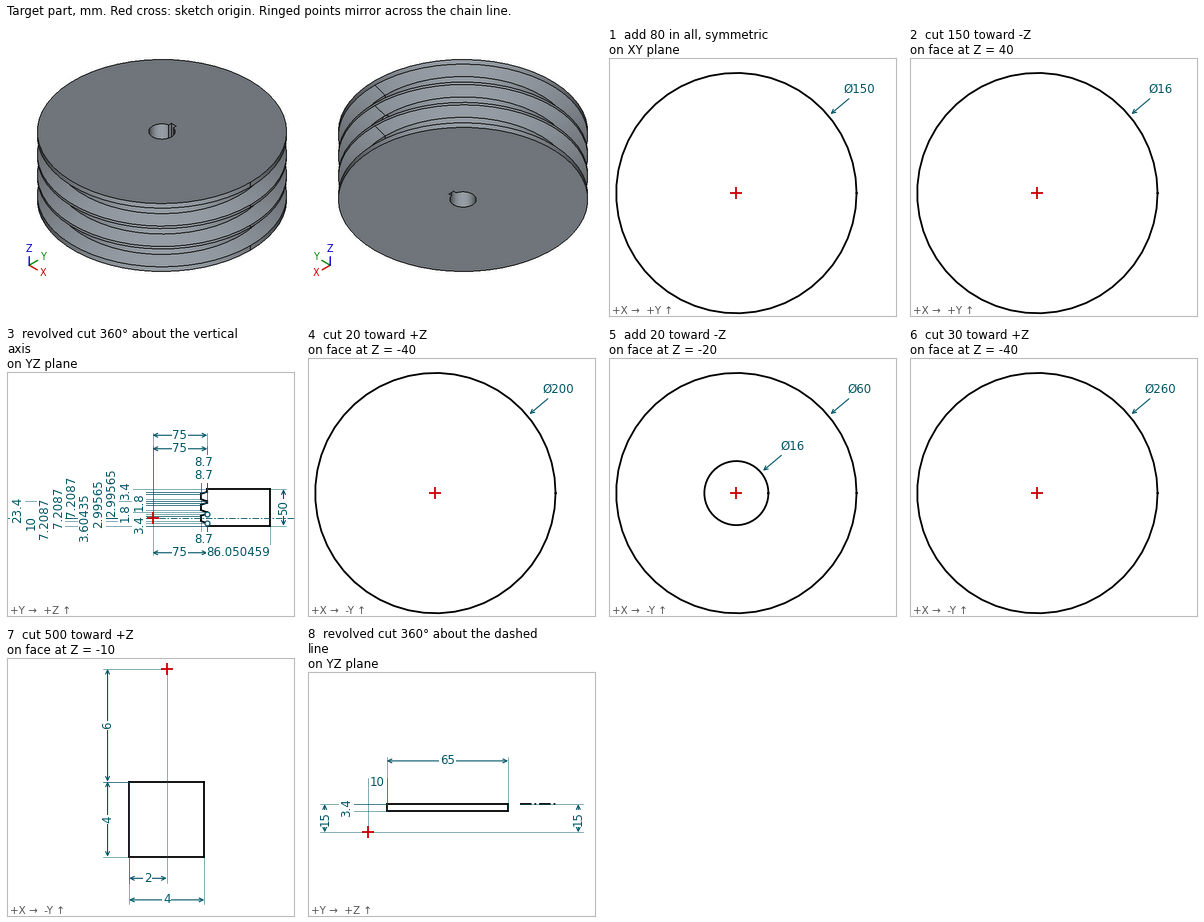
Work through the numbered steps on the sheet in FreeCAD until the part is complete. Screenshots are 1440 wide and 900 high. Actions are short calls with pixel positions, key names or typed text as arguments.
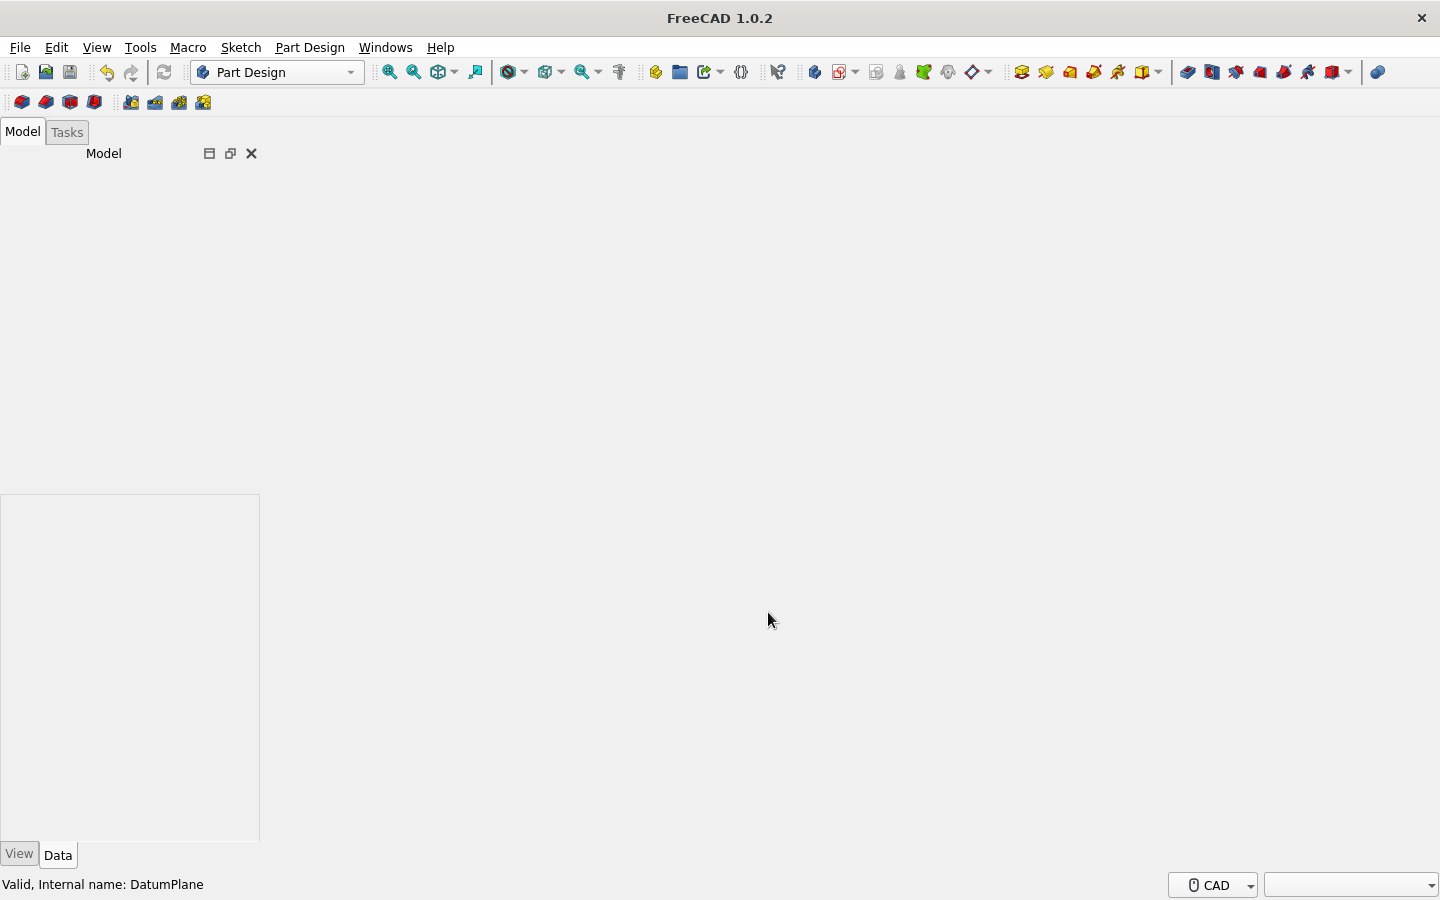
key(ctrl+n)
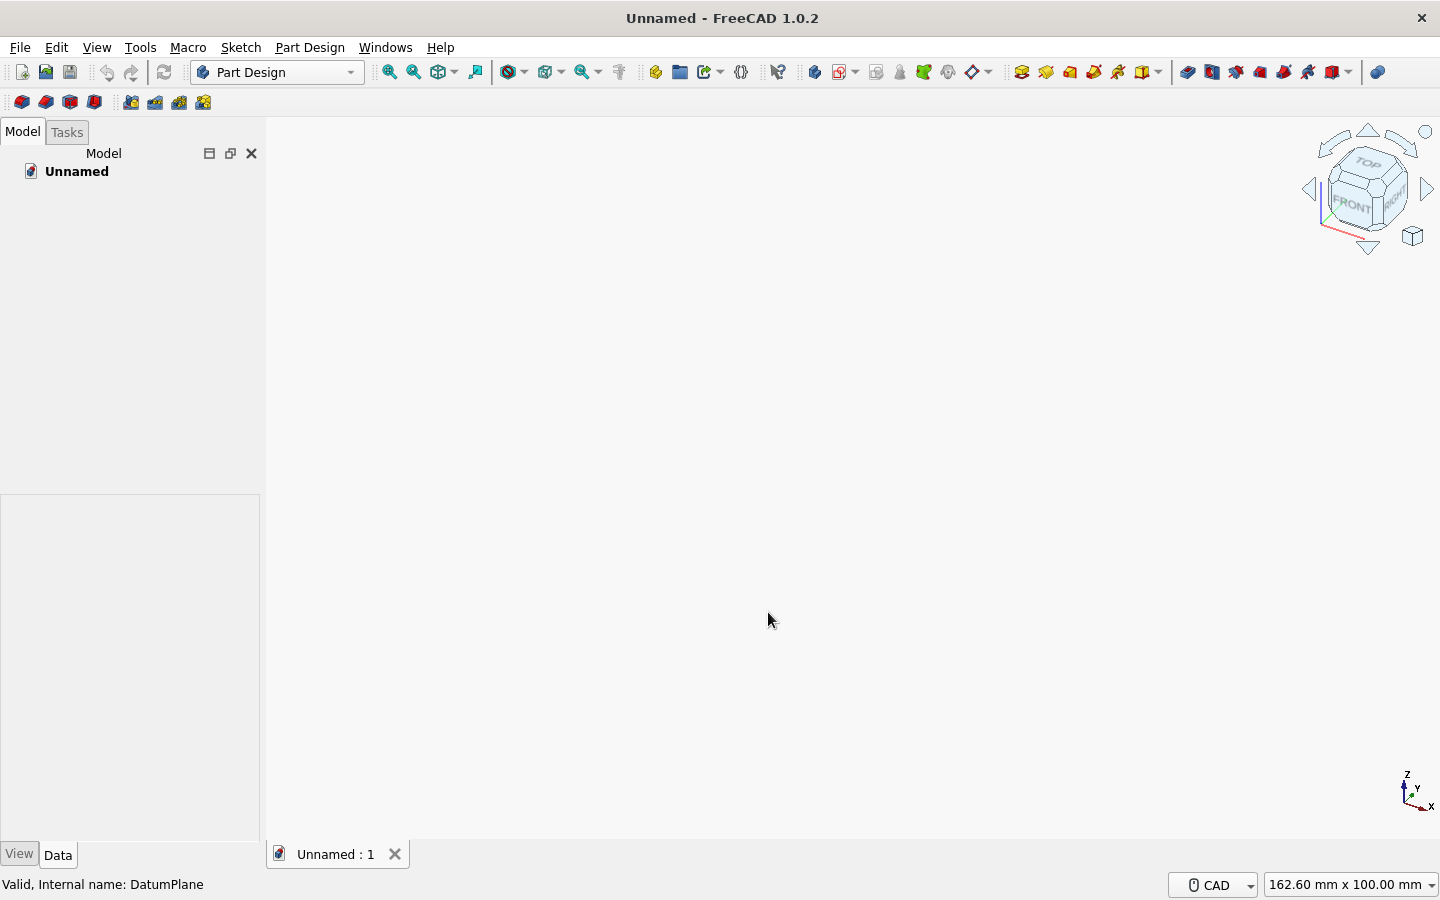
click(840, 72)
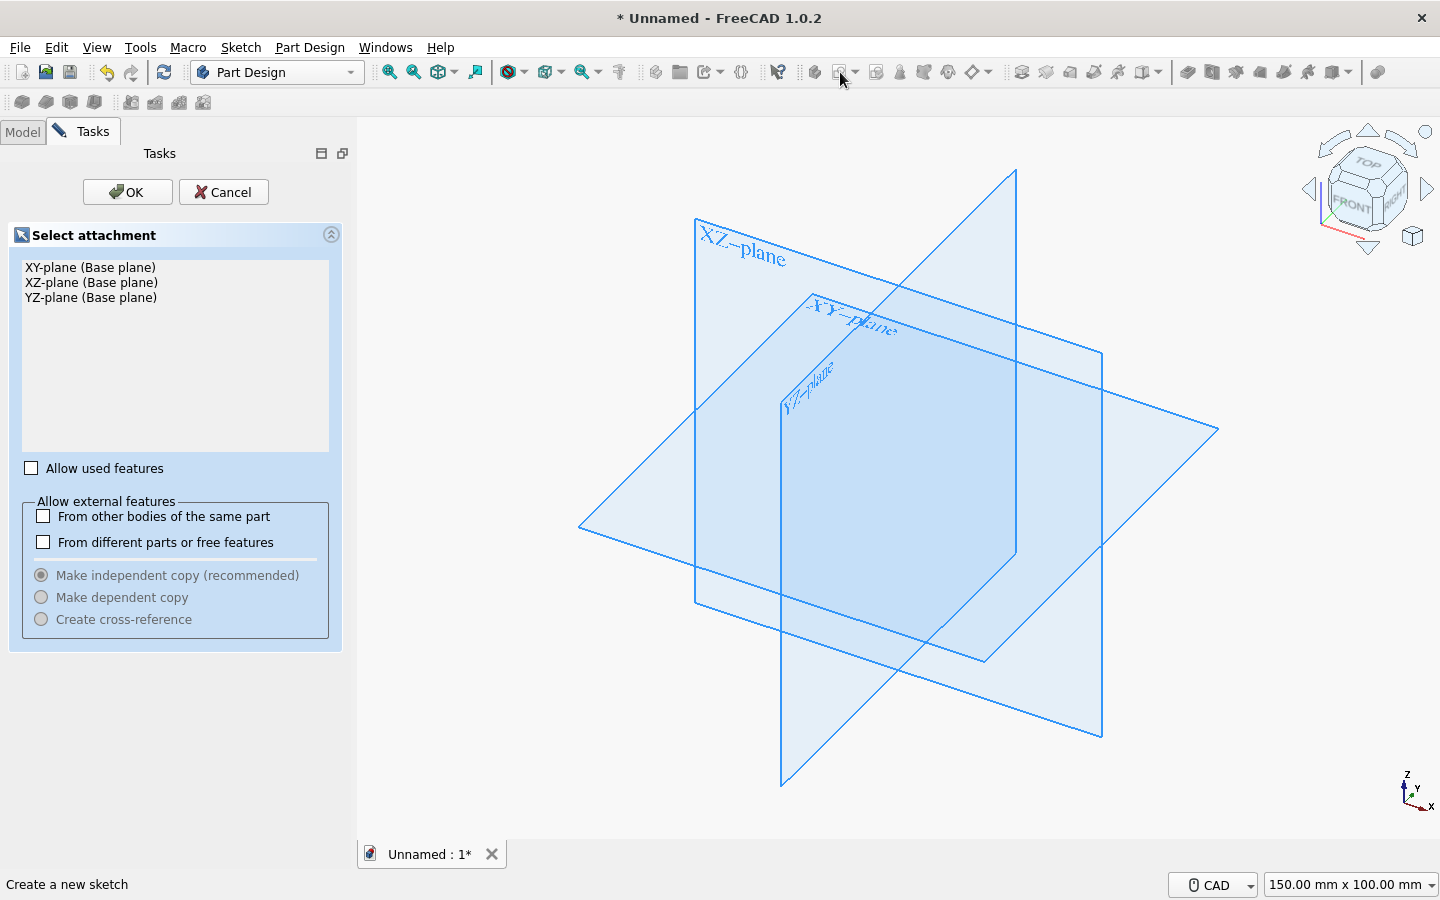
click(82, 268)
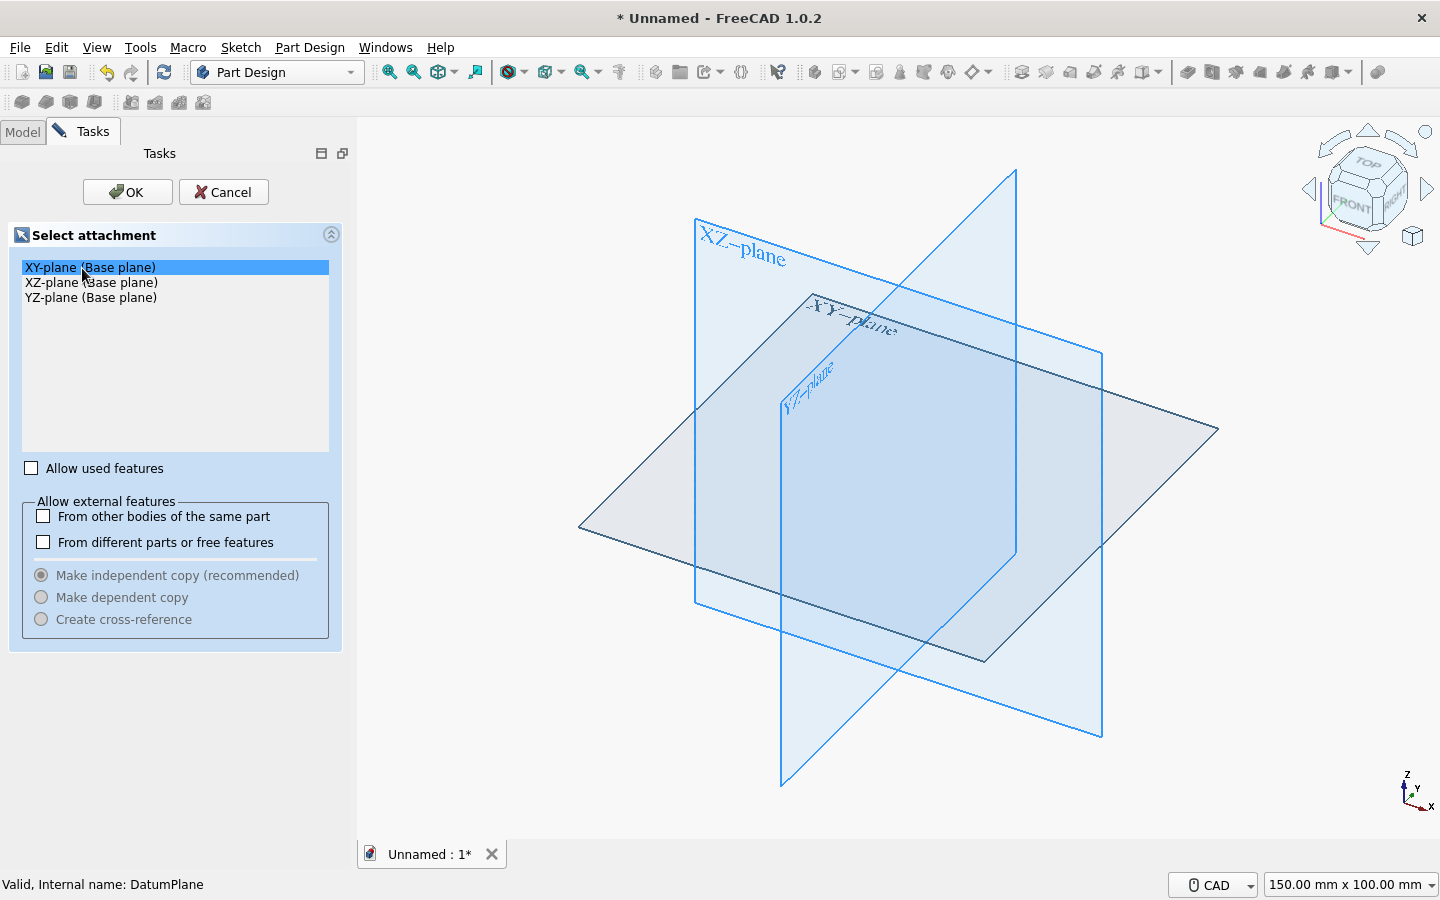
click(128, 192)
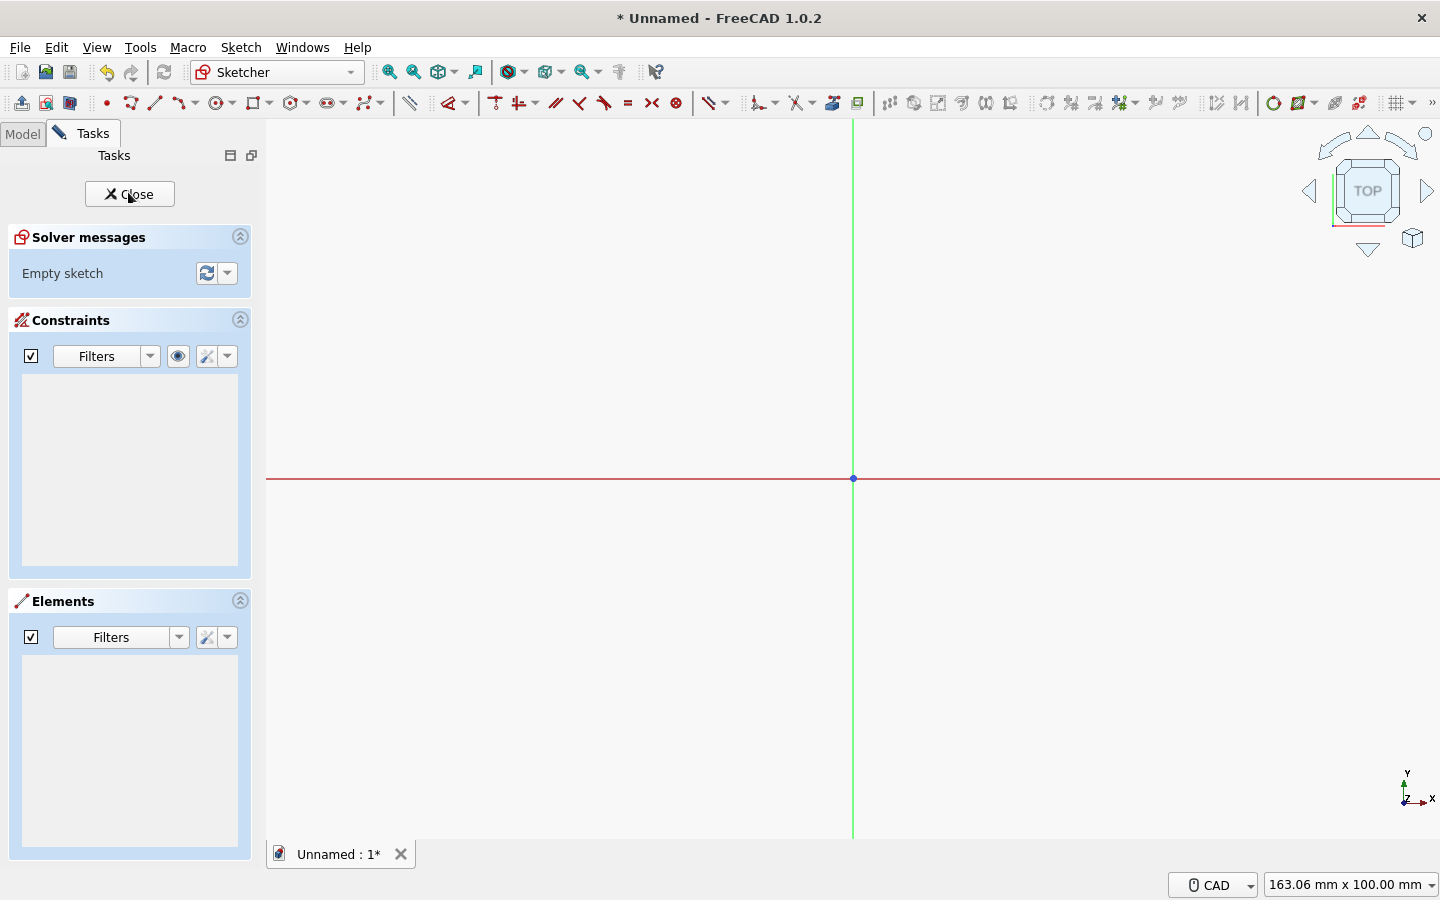
scroll(729, 479, down, 4)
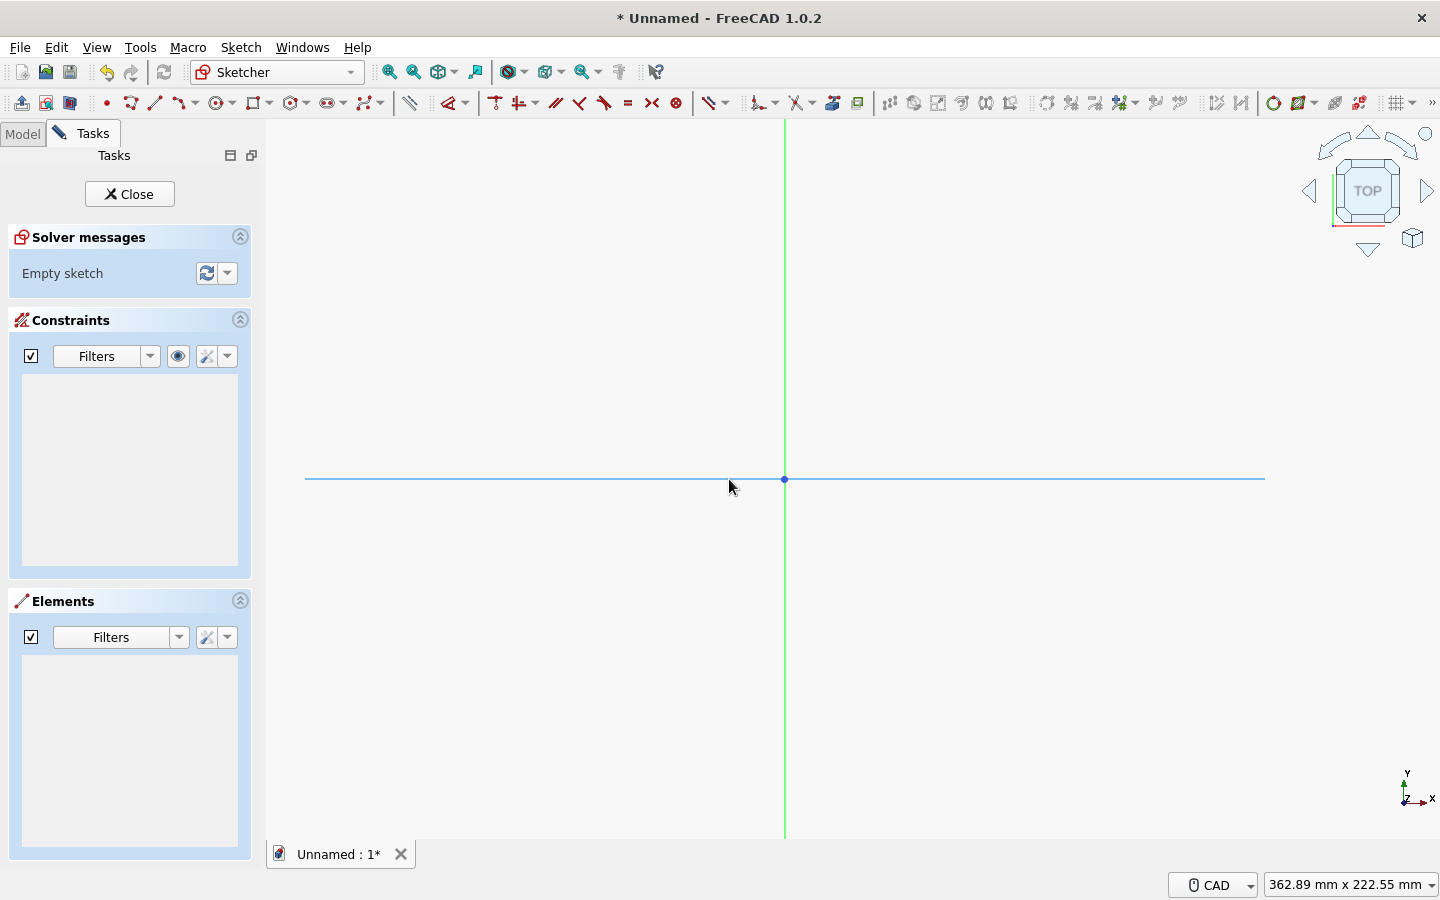
click(216, 104)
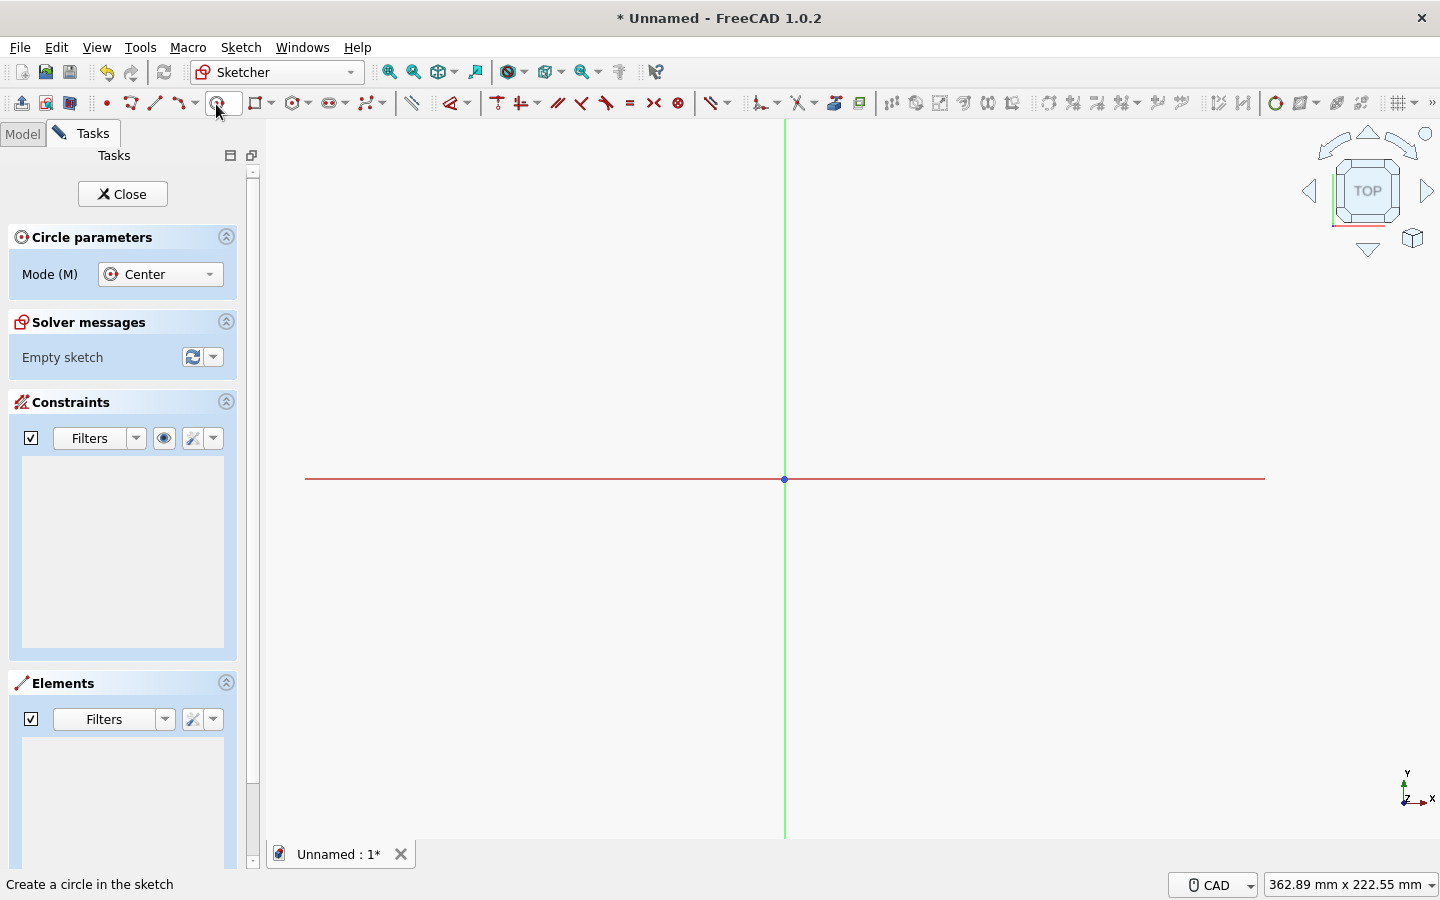
click(785, 479)
click(957, 308)
key(Escape)